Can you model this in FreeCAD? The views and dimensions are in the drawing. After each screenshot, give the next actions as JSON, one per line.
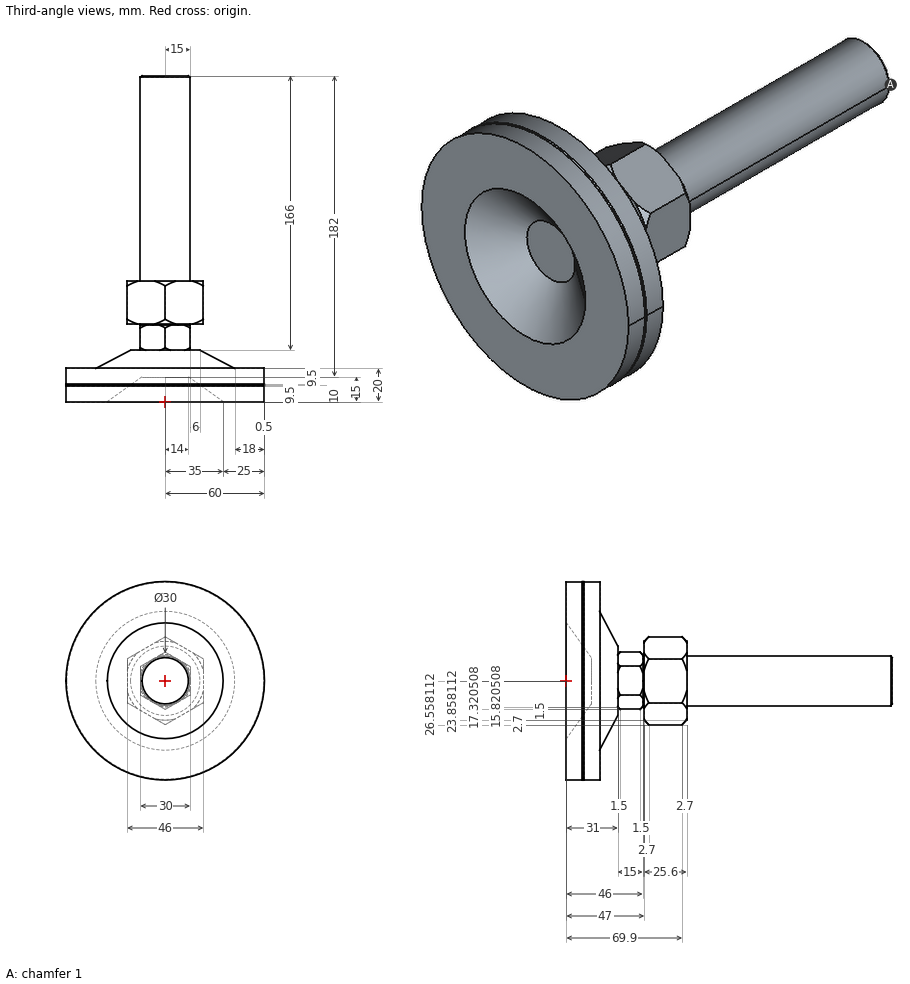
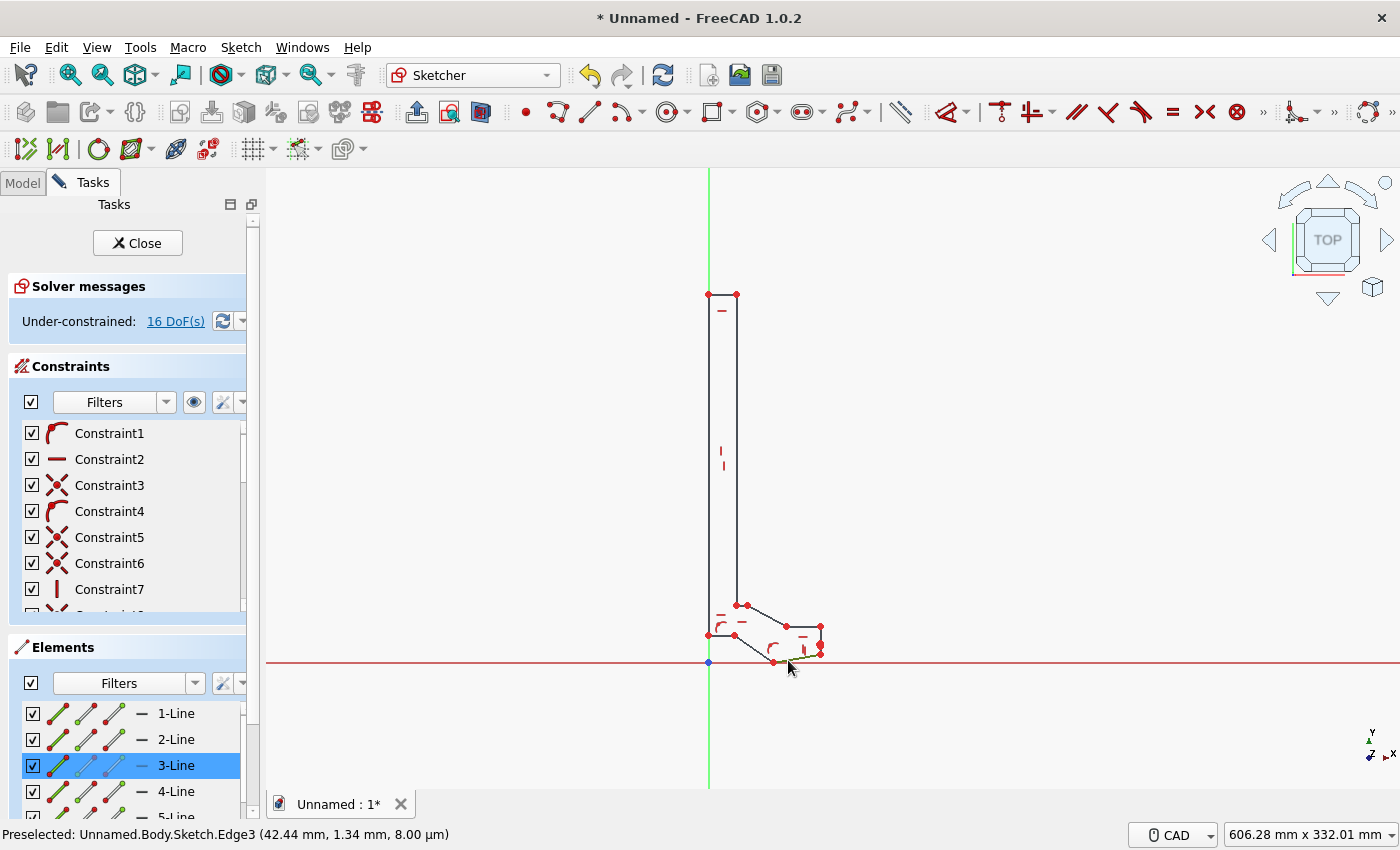
{"action": "key", "text": "h"}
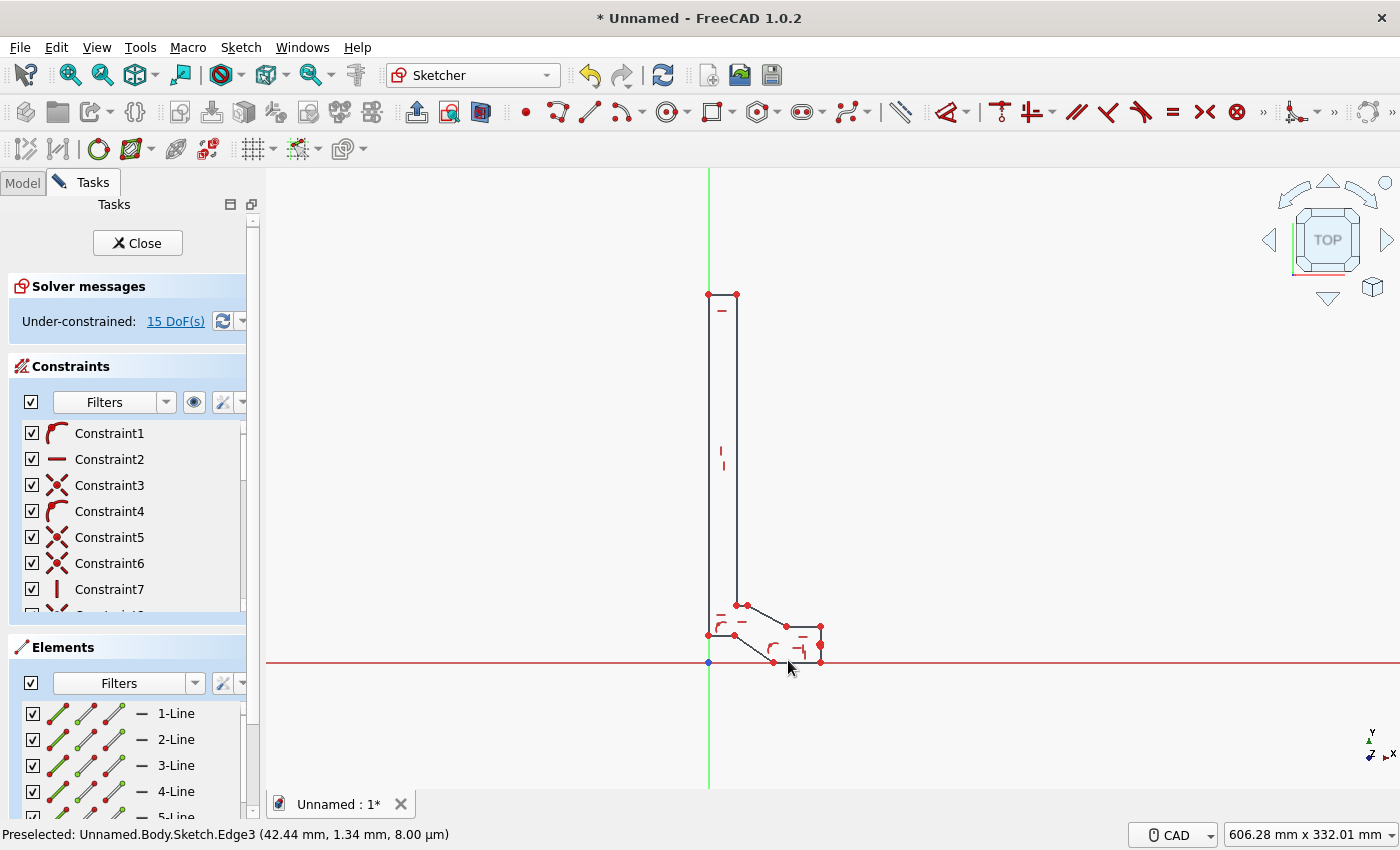
{"action": "scroll", "coordinate": [742, 606], "scroll_direction": "up", "scroll_amount": 7}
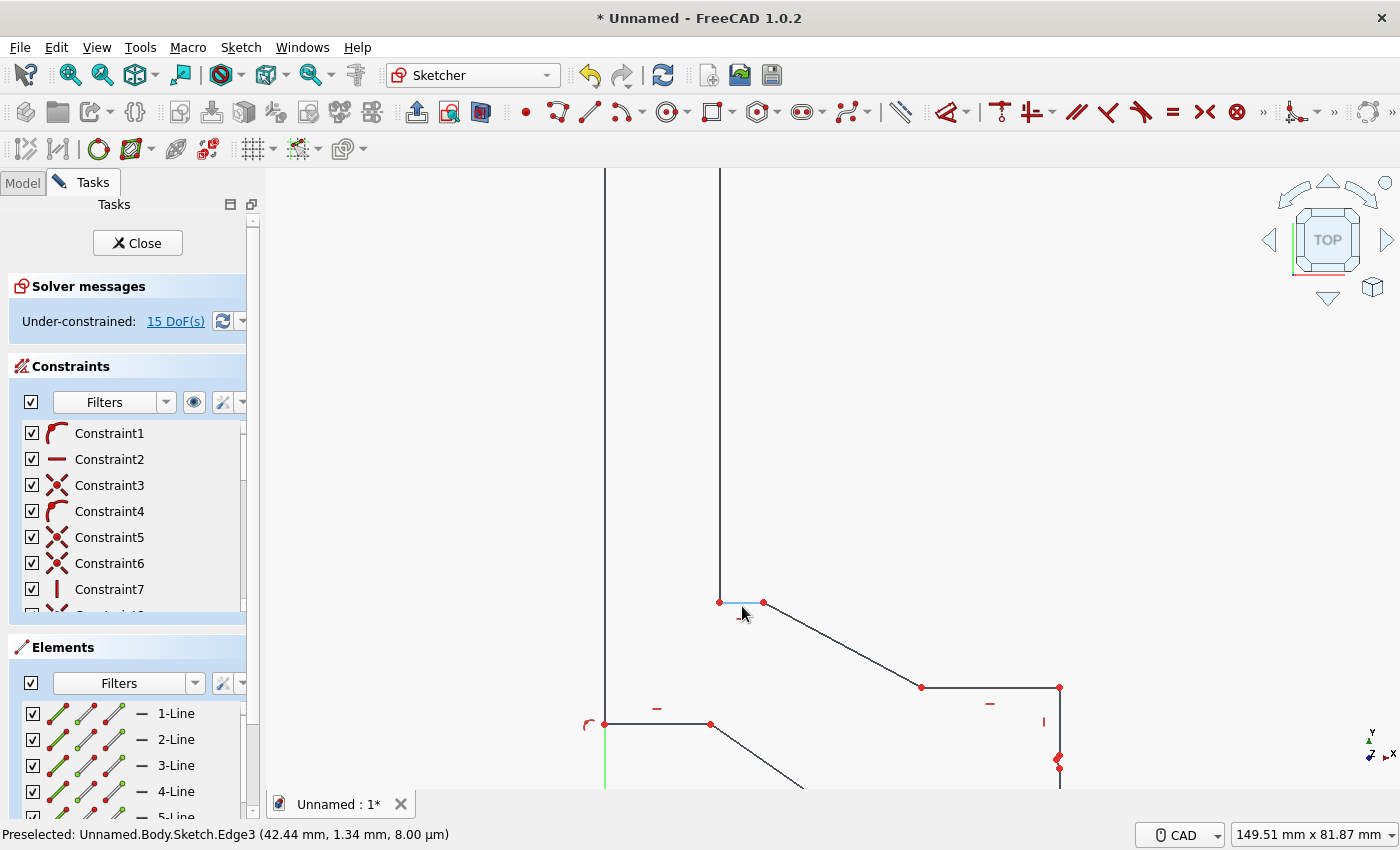
{"action": "left_click", "coordinate": [742, 603]}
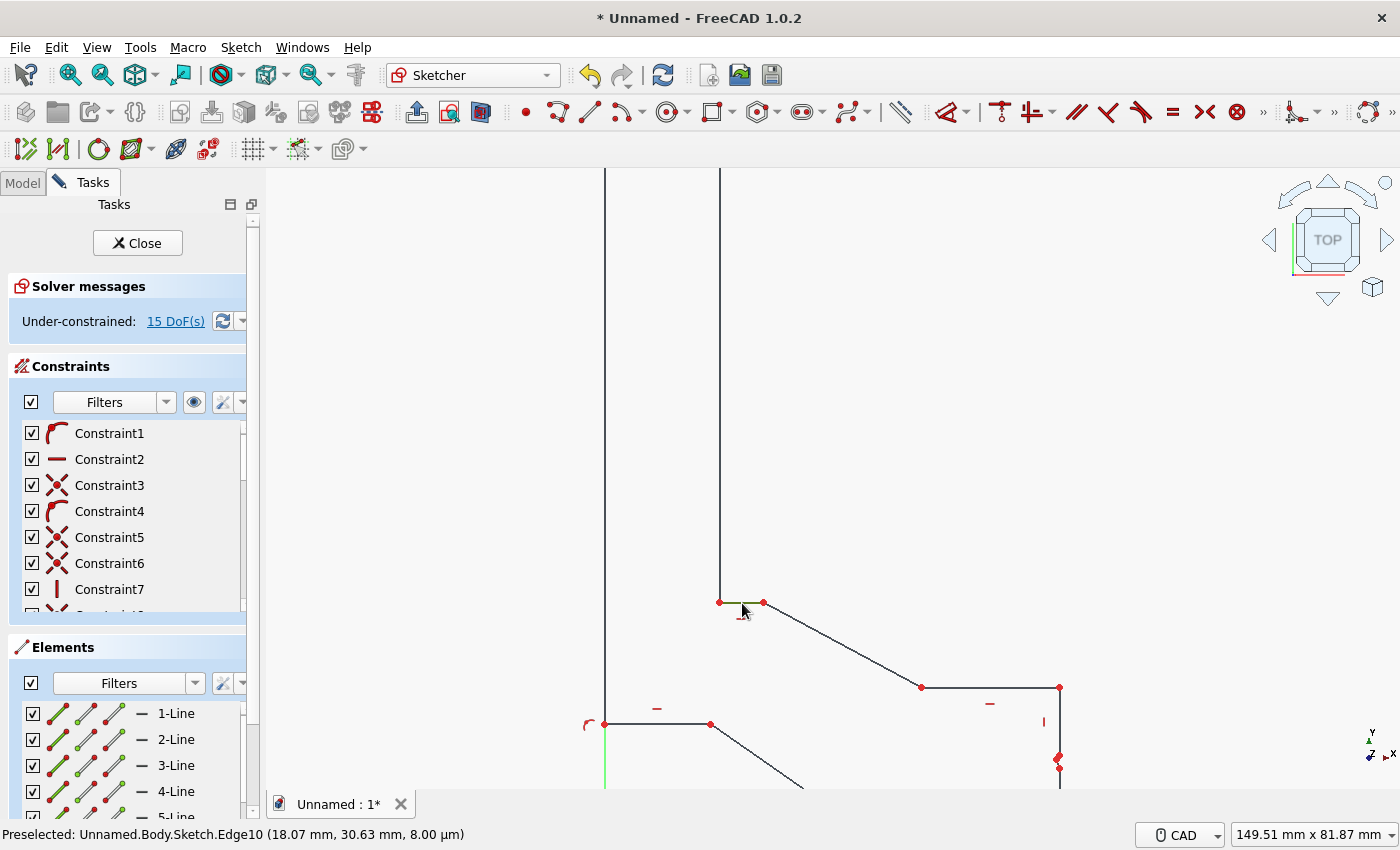
{"action": "key", "text": "l"}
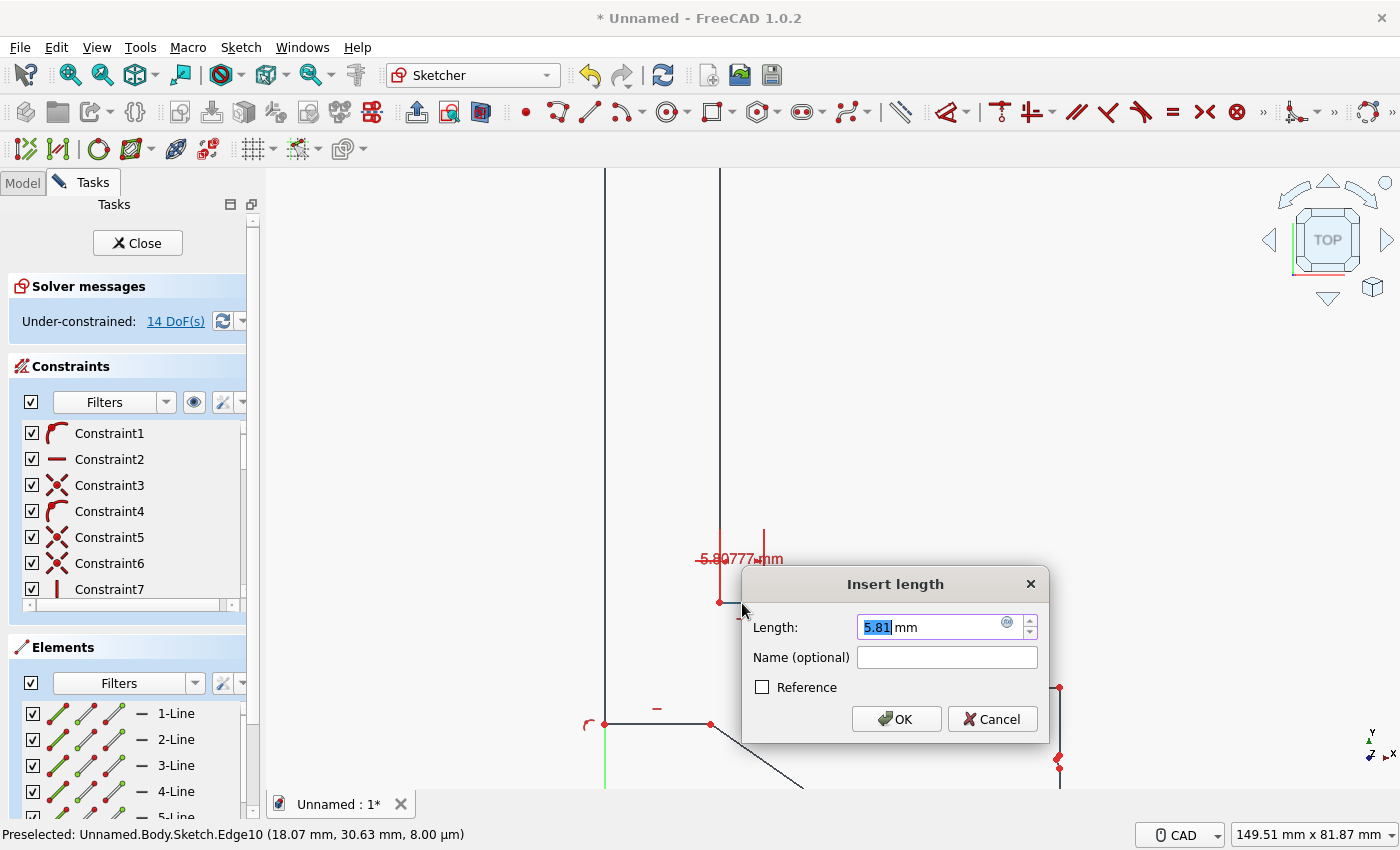
{"action": "type", "text": "6"}
{"action": "key", "text": "Return"}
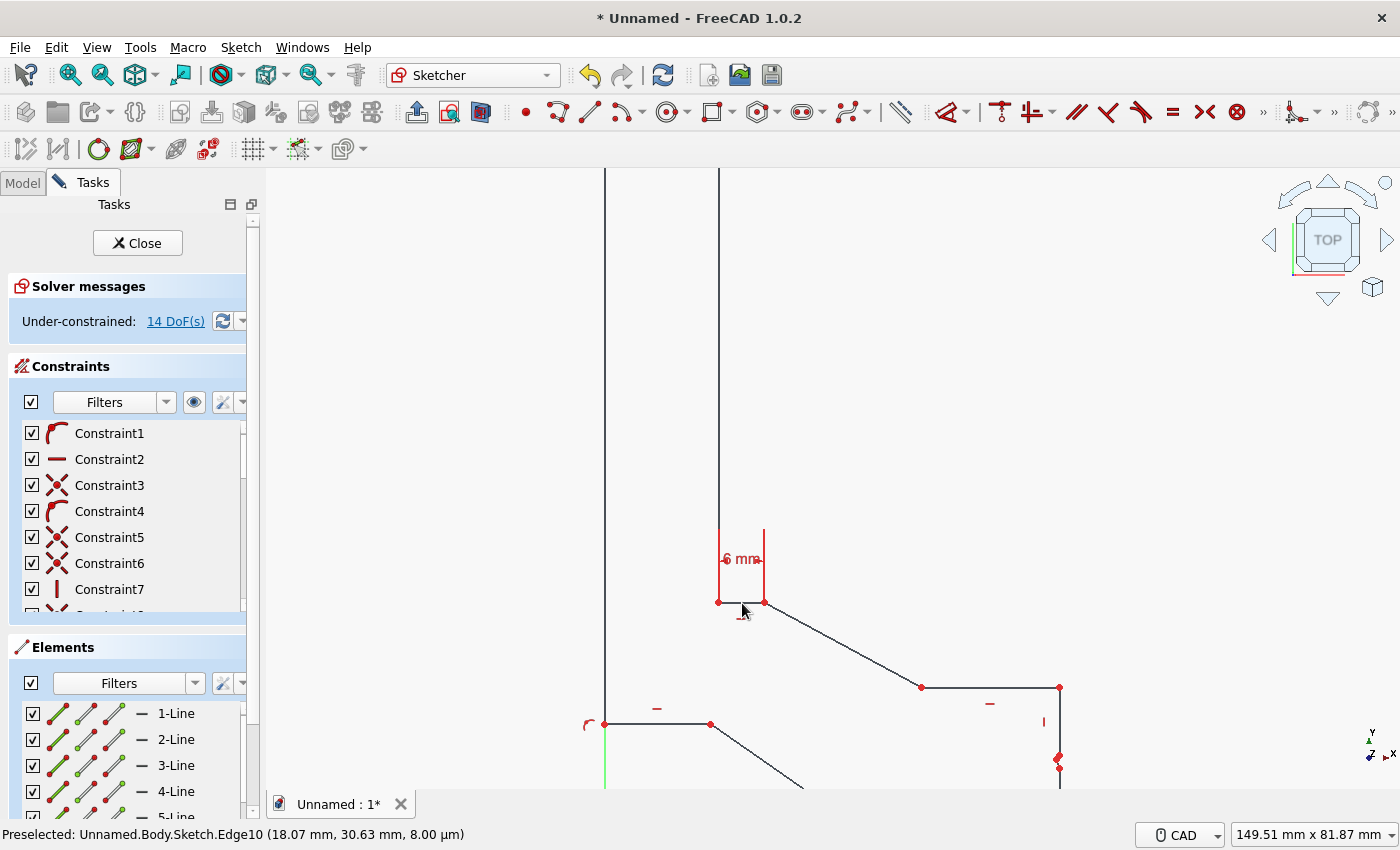
{"action": "left_click", "coordinate": [637, 724]}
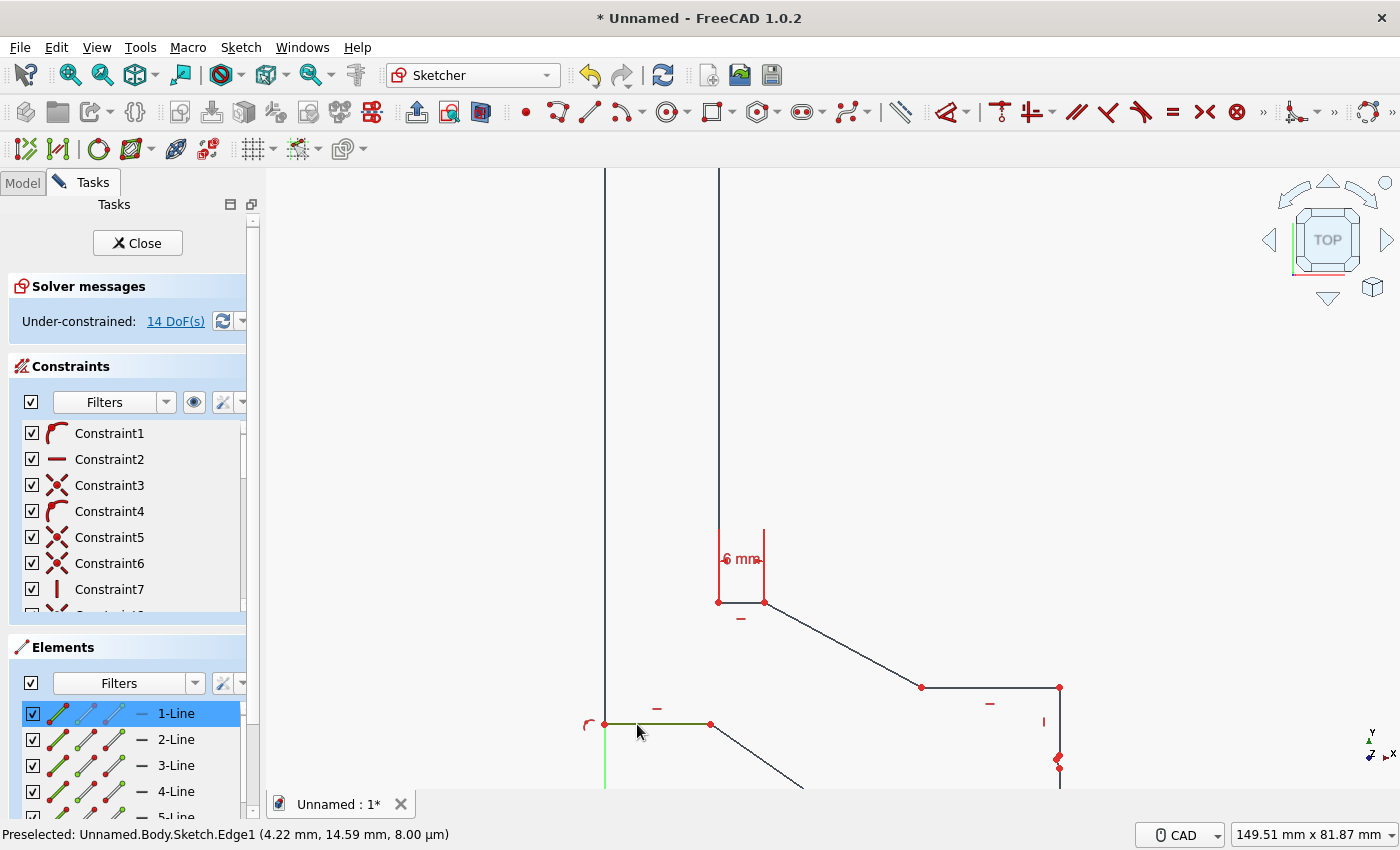
{"action": "key", "text": "l"}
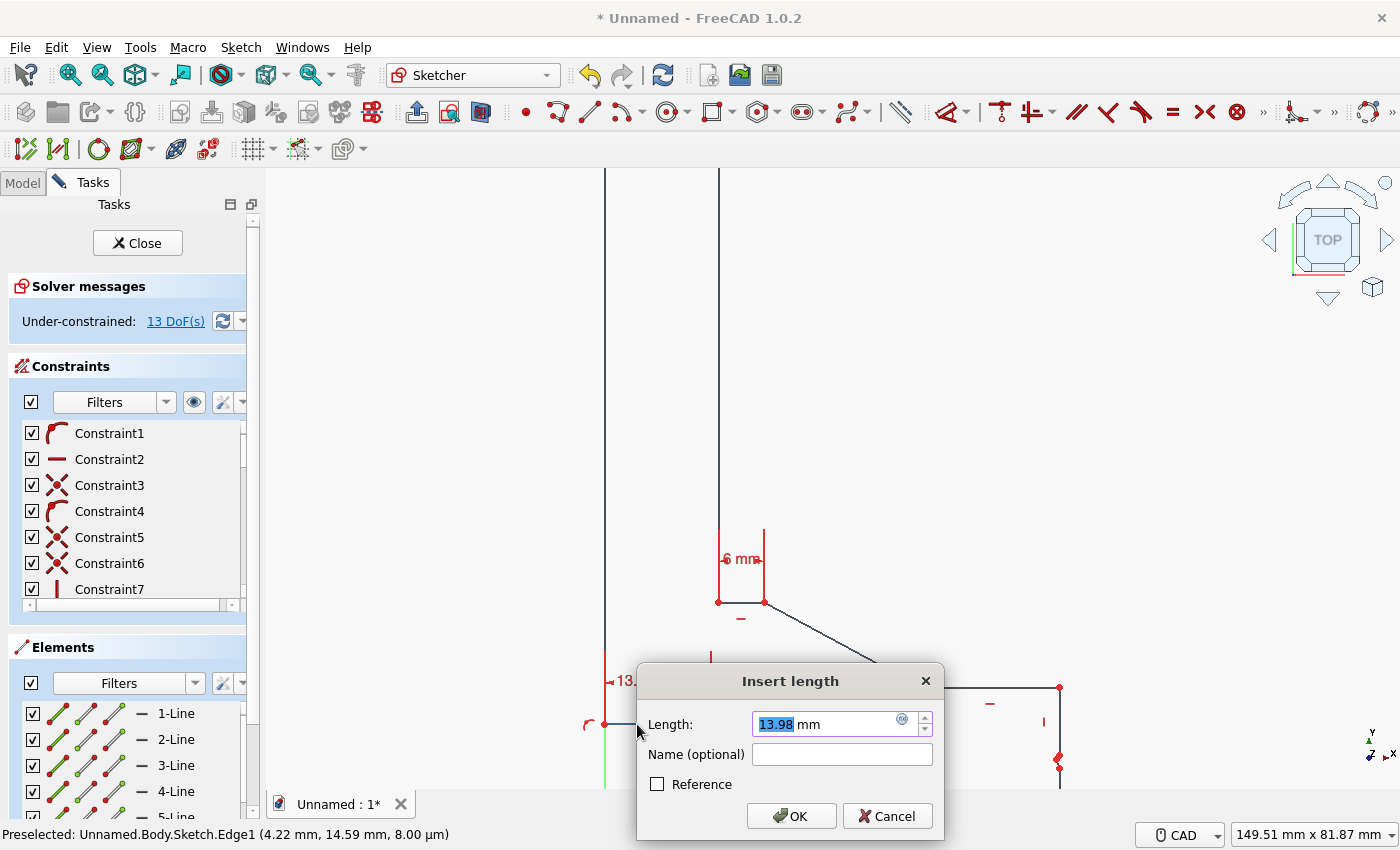
{"action": "type", "text": "14"}
{"action": "key", "text": "Return"}